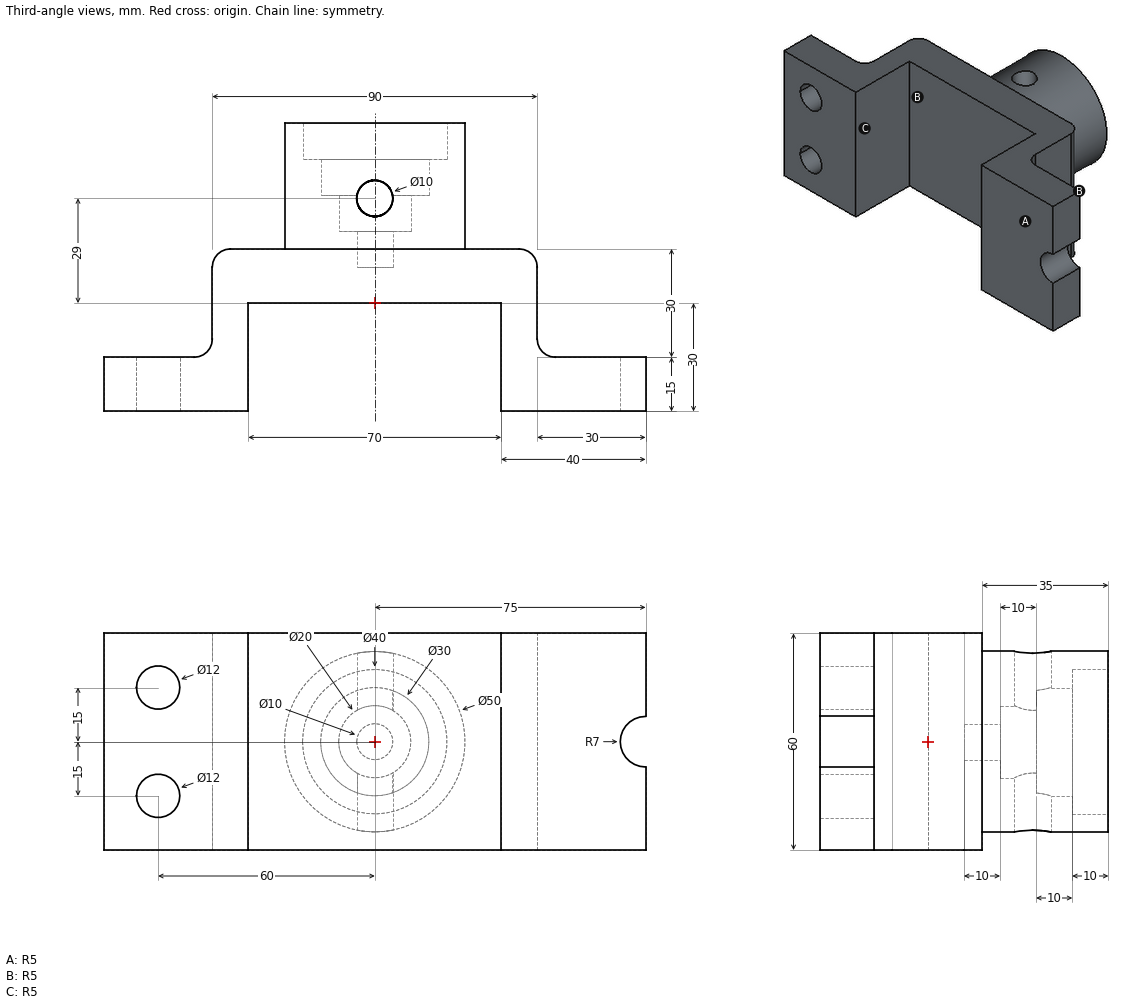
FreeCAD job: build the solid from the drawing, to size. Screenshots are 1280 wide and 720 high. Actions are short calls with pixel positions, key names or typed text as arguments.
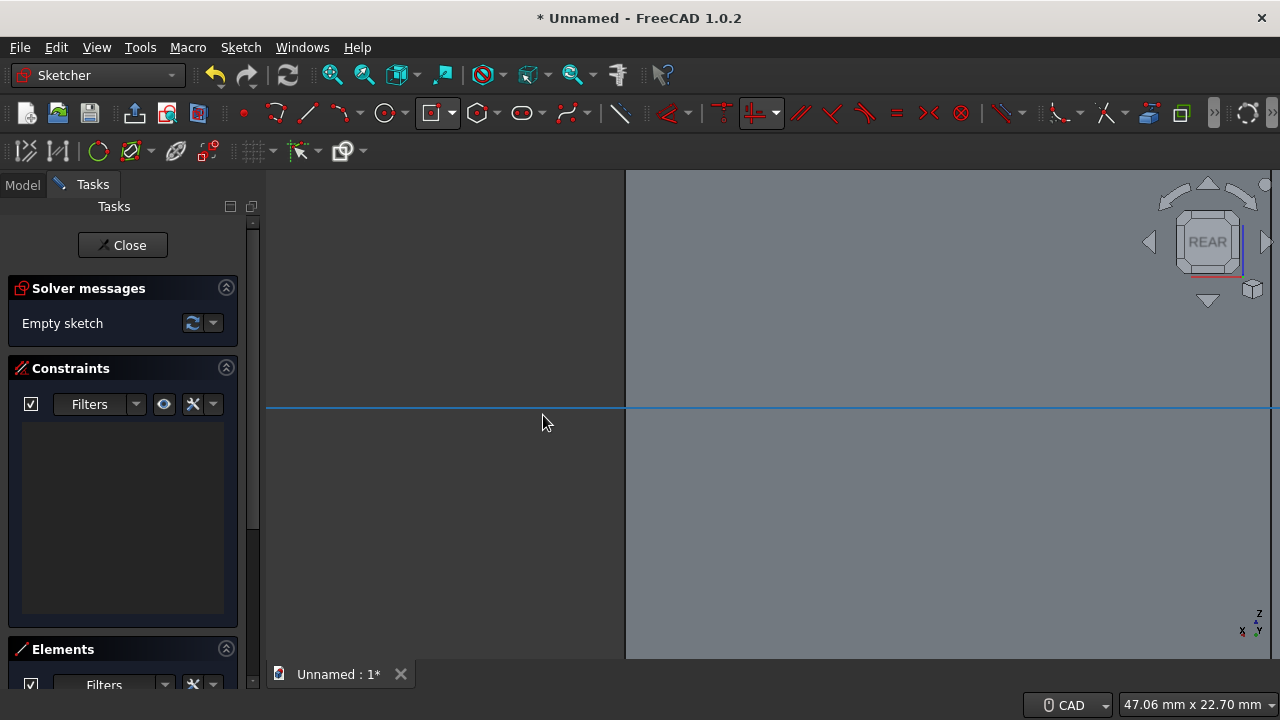
key(g)
key(l)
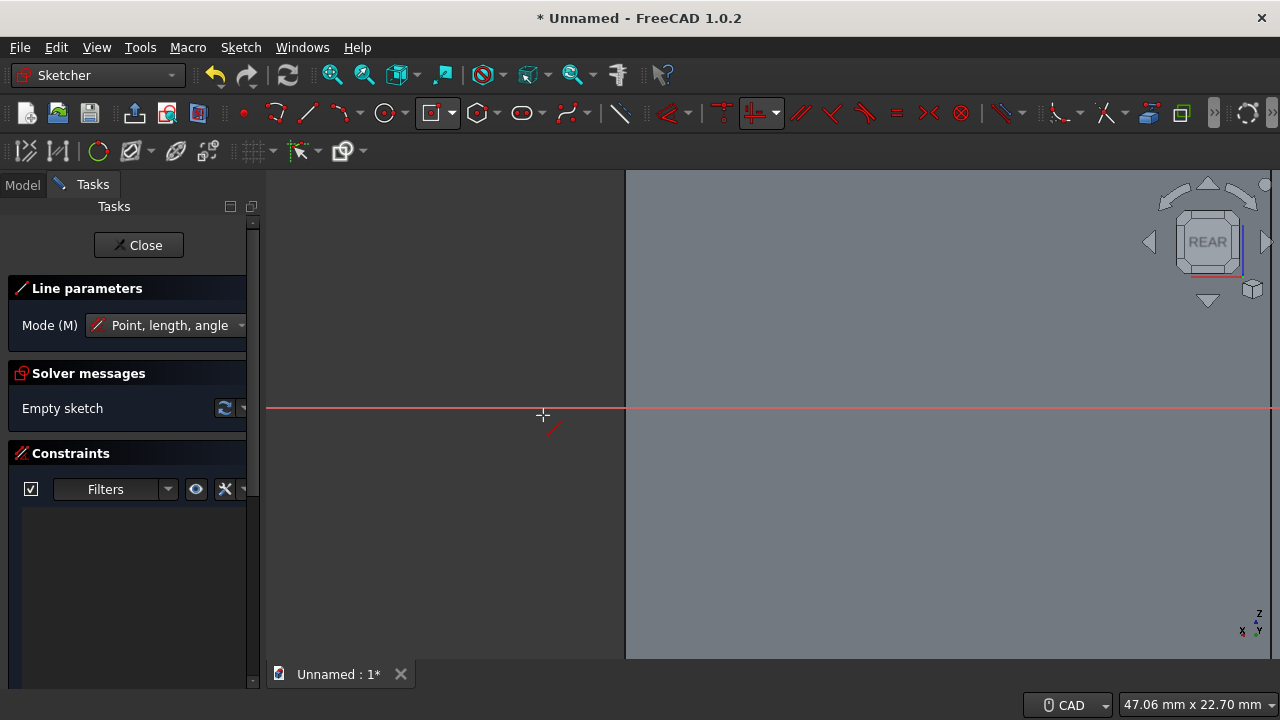
click(625, 257)
click(625, 559)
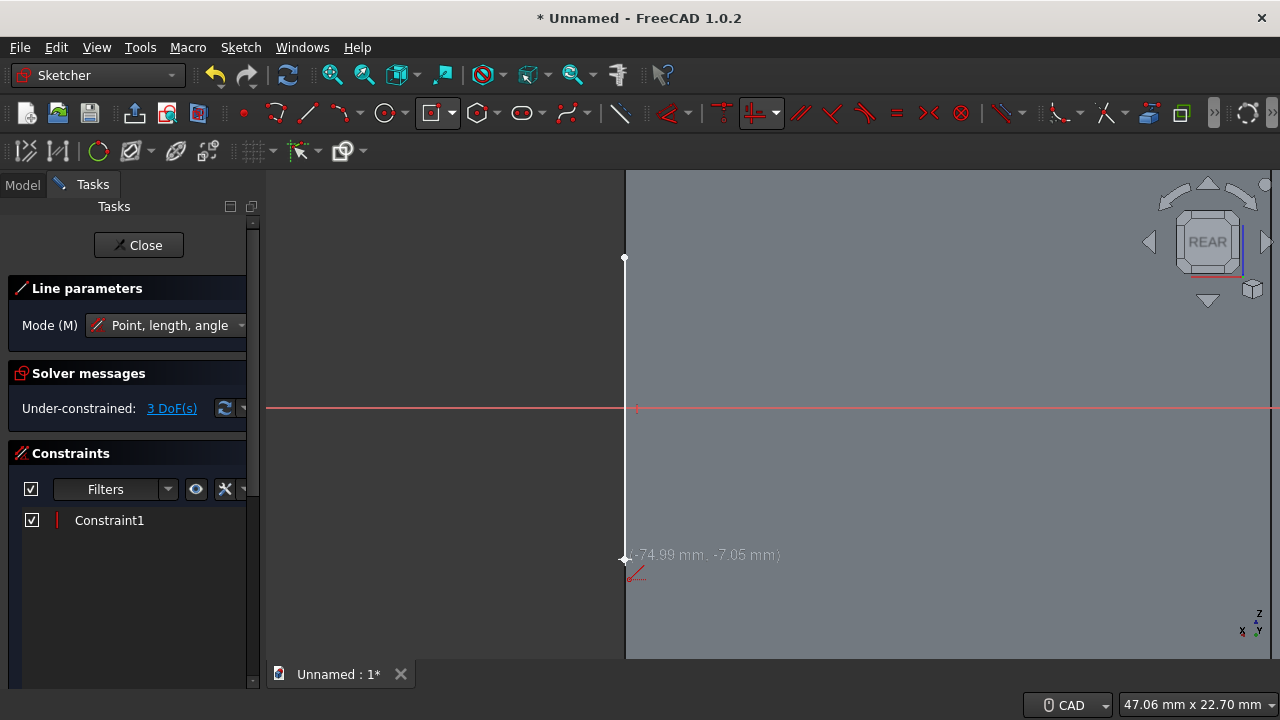
click(340, 114)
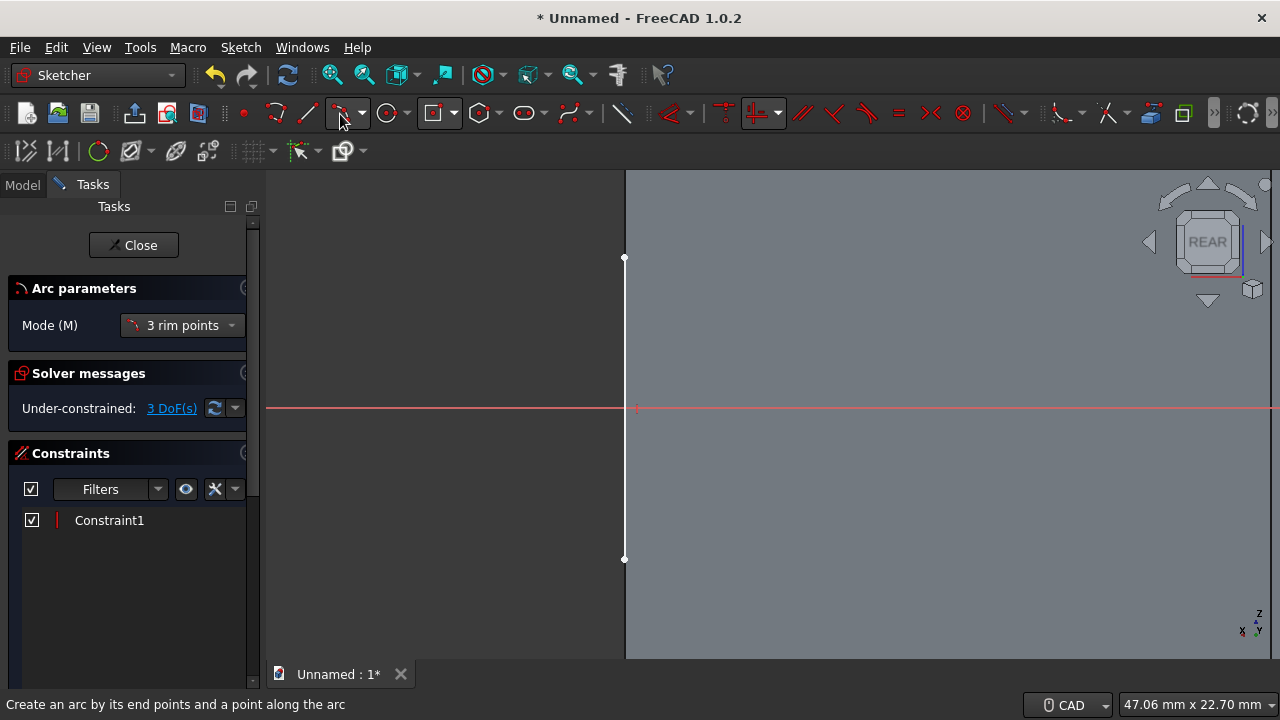
click(625, 560)
click(625, 258)
click(768, 455)
key(Escape)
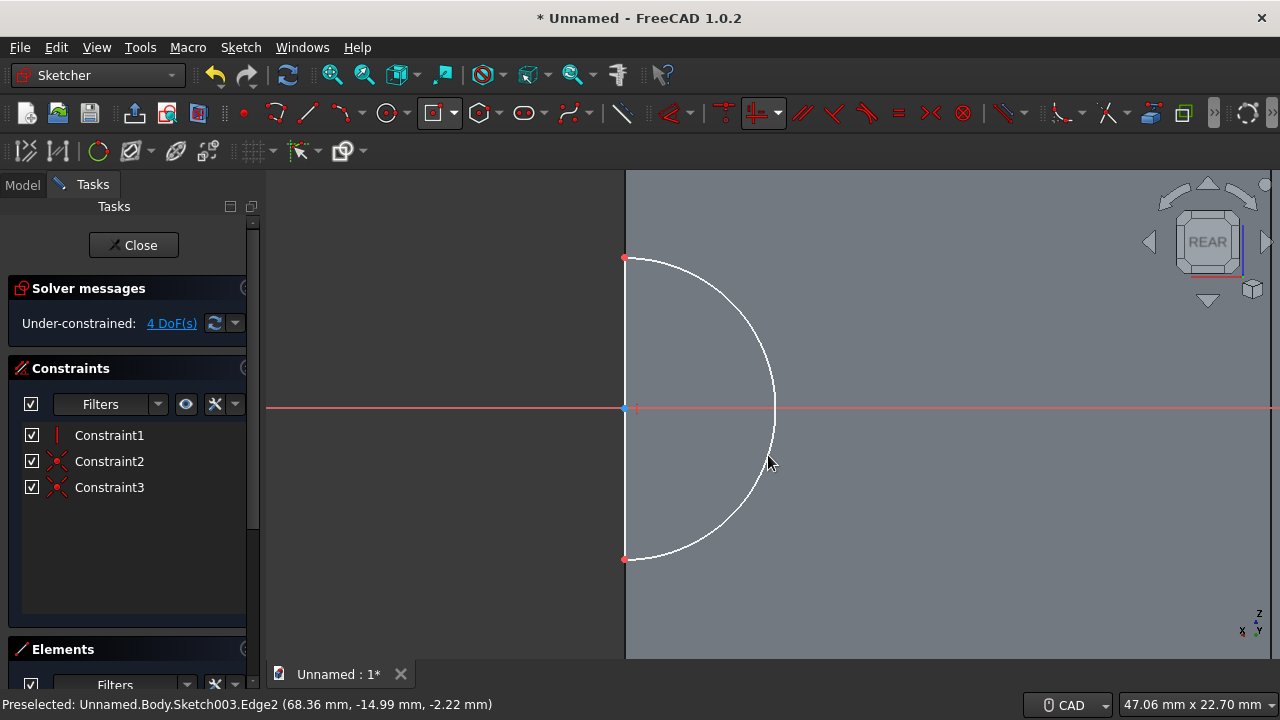
click(624, 409)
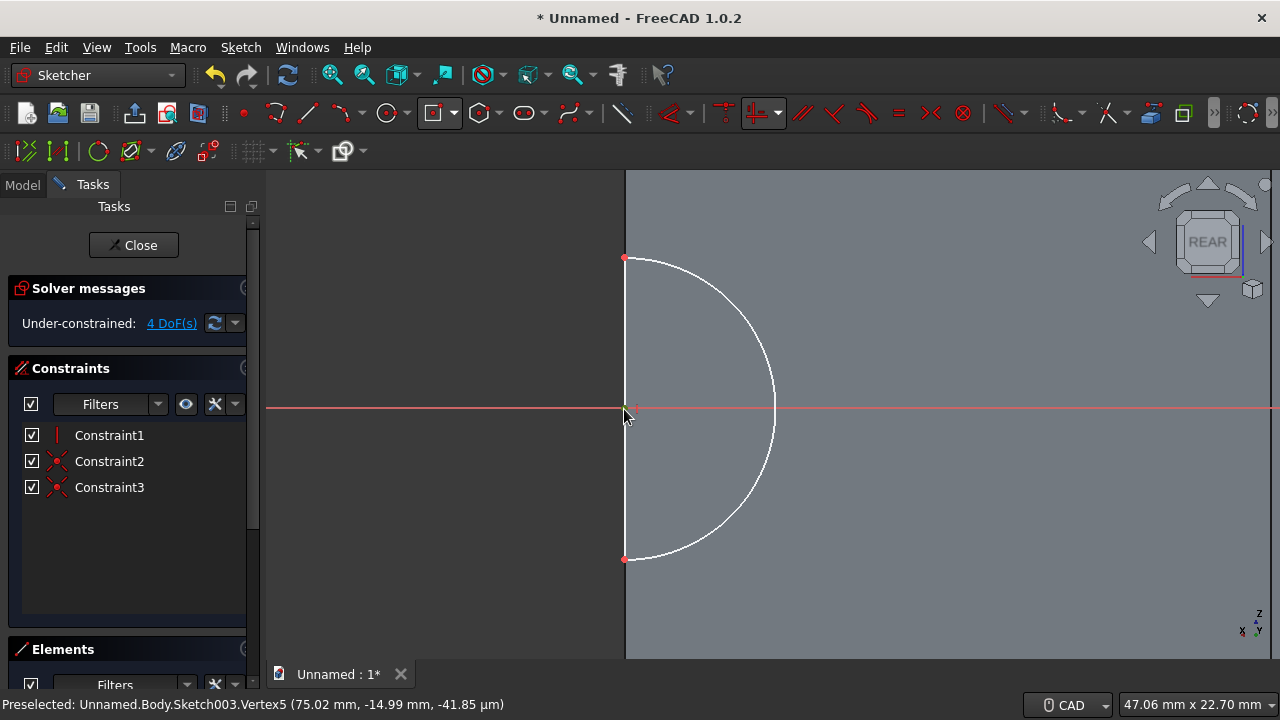
click(353, 408)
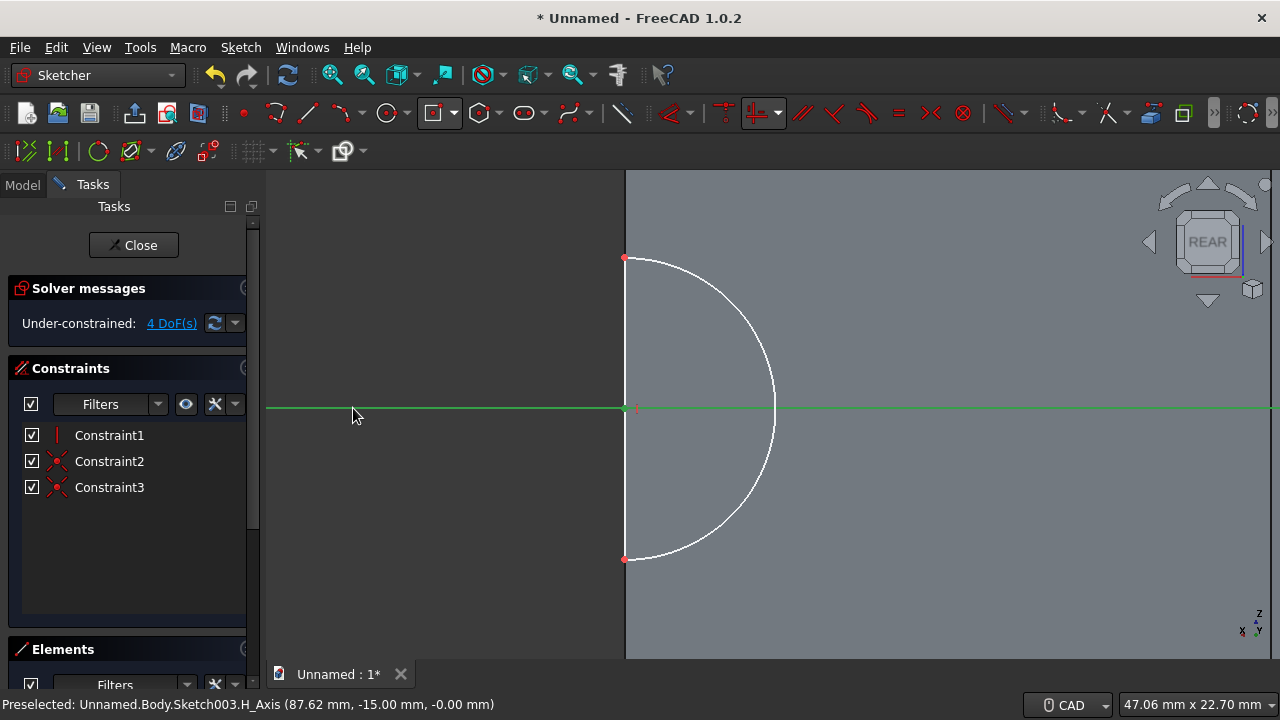
click(724, 114)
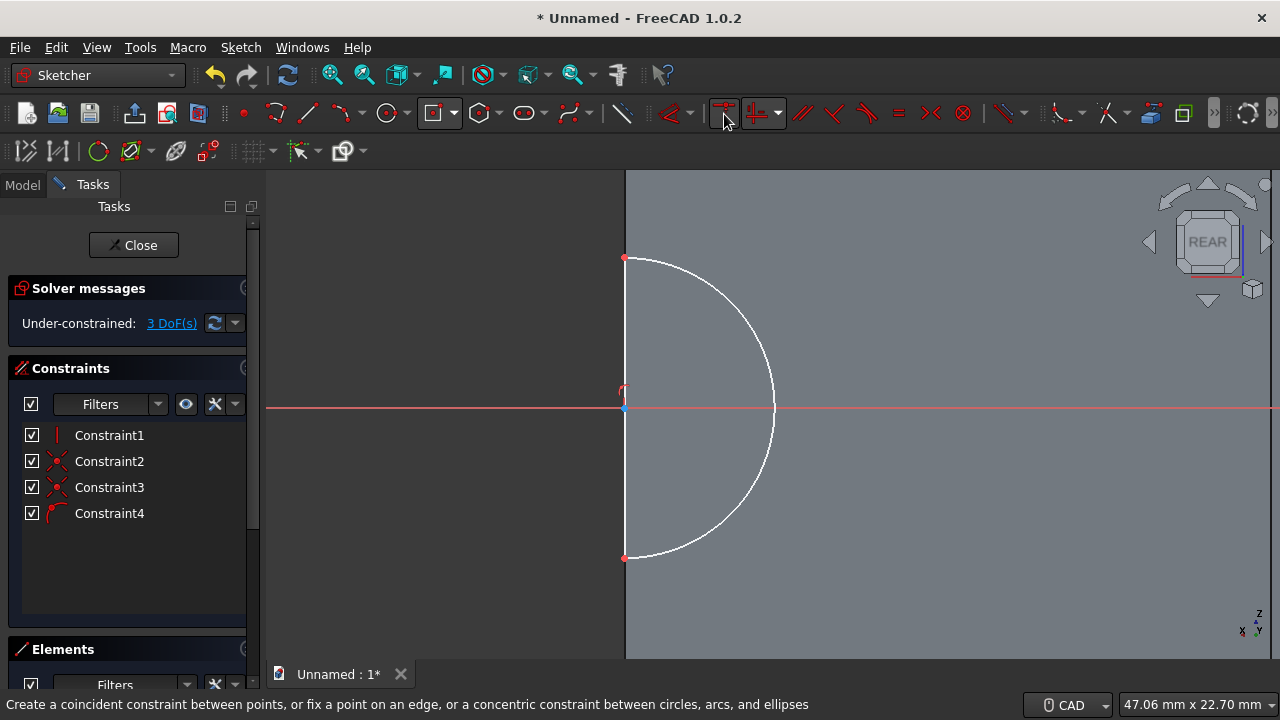
click(670, 114)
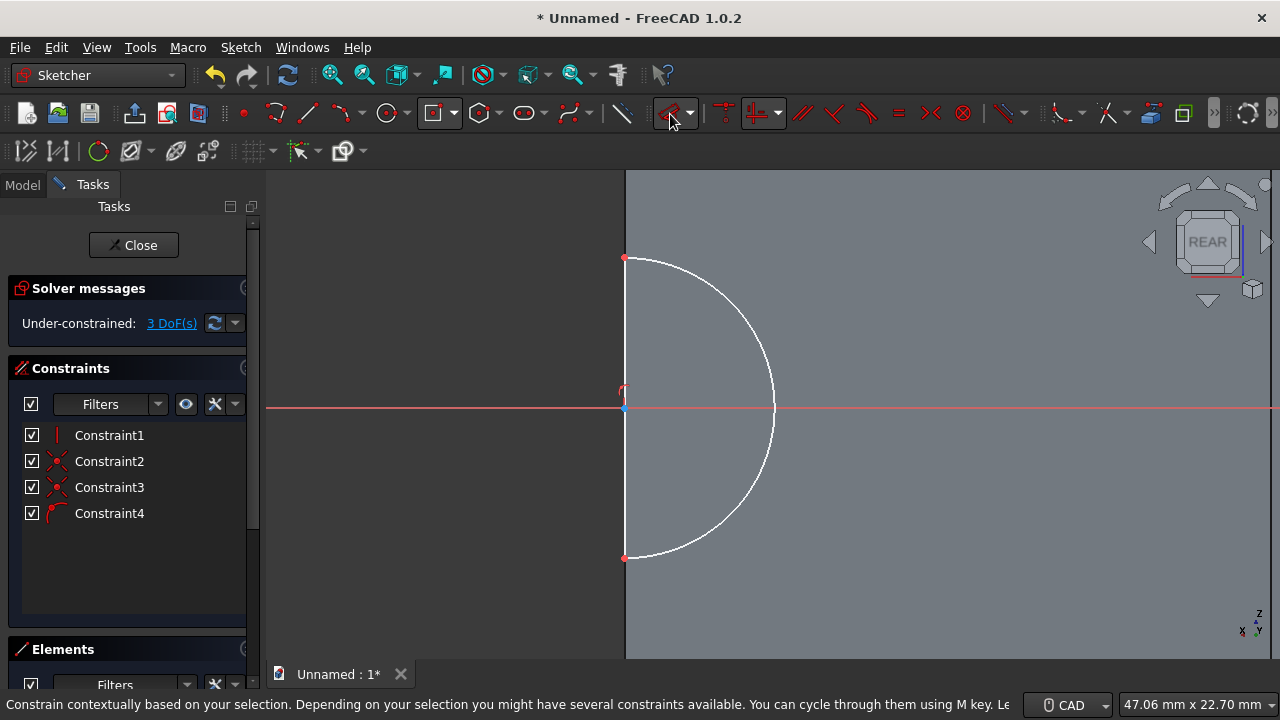
click(746, 496)
click(772, 515)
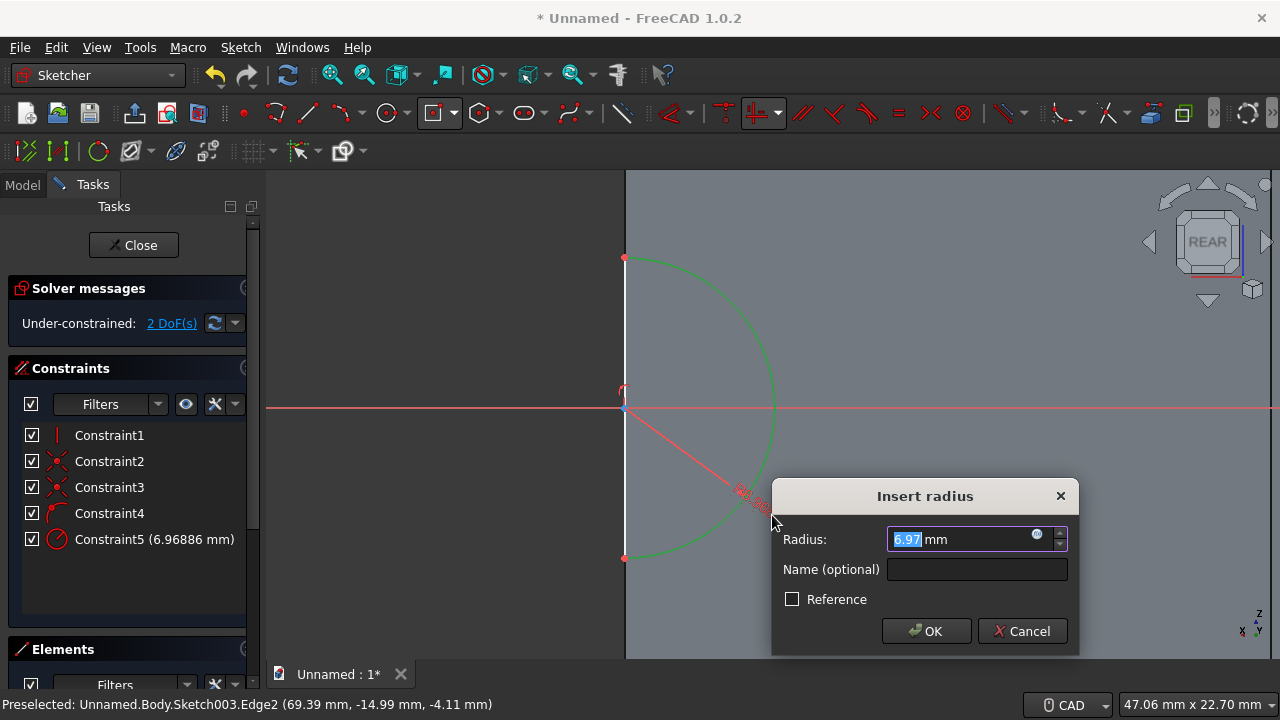
text(7)
key(Return)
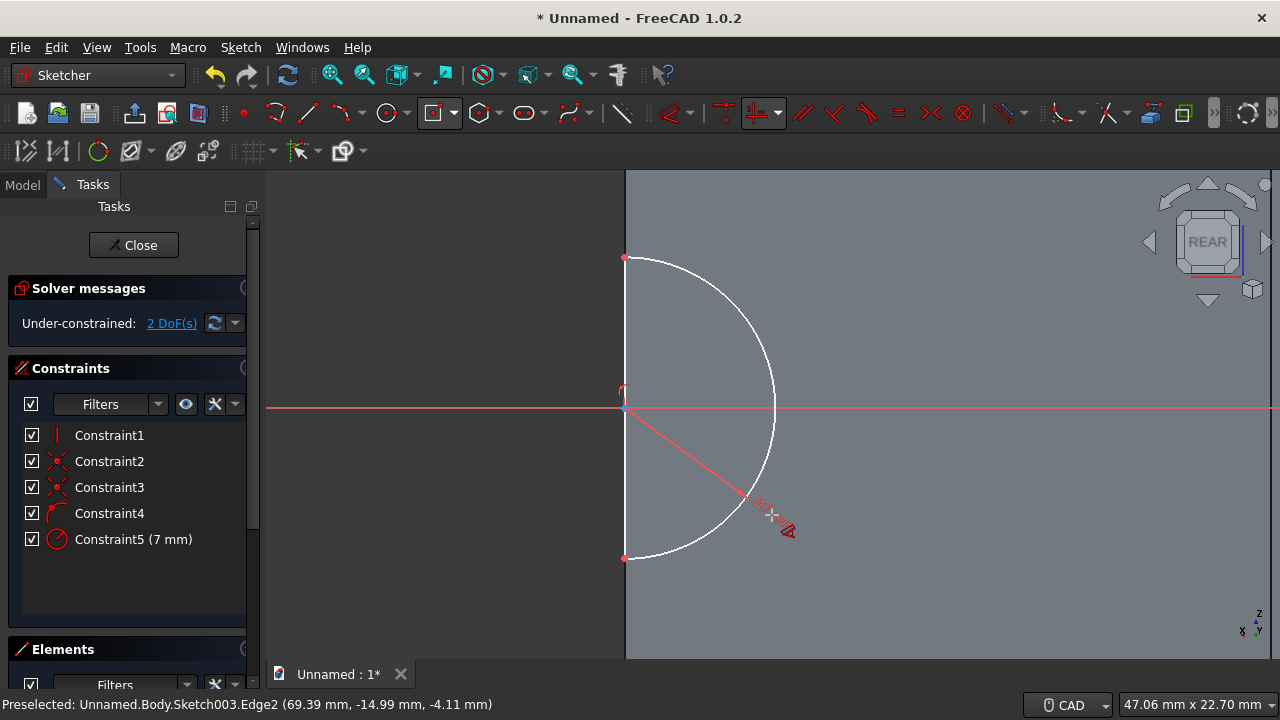
click(625, 257)
click(870, 223)